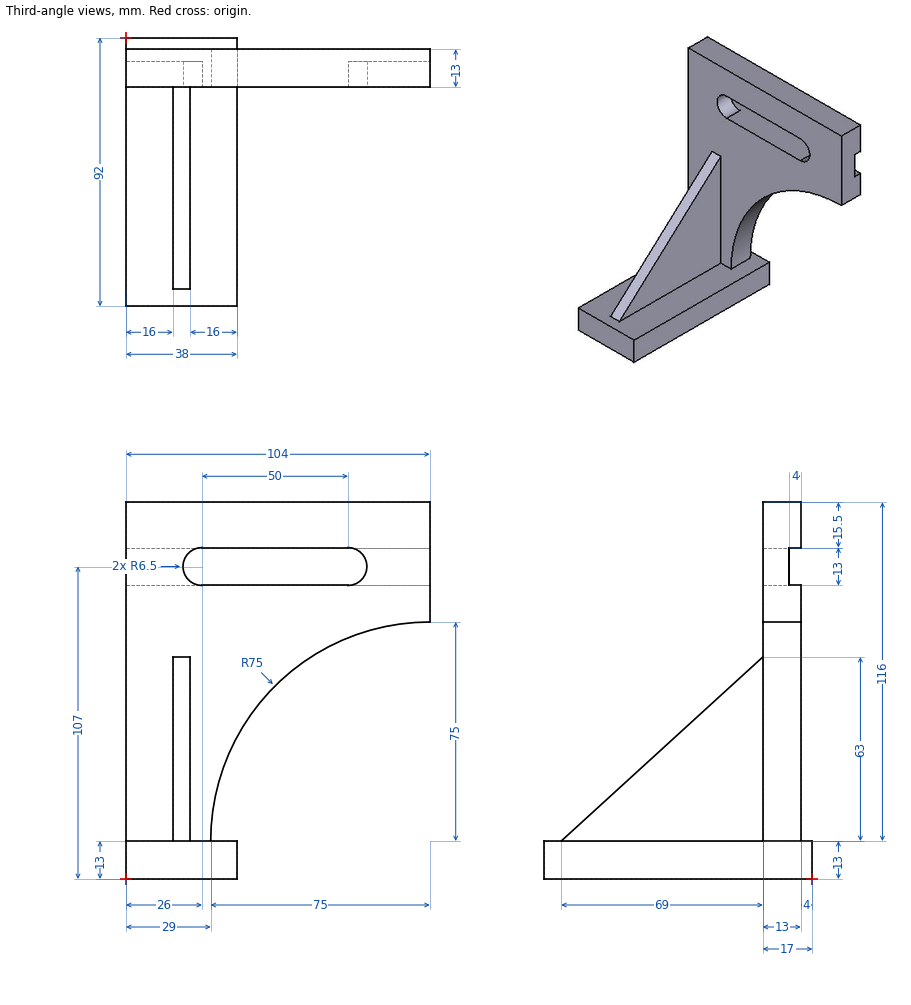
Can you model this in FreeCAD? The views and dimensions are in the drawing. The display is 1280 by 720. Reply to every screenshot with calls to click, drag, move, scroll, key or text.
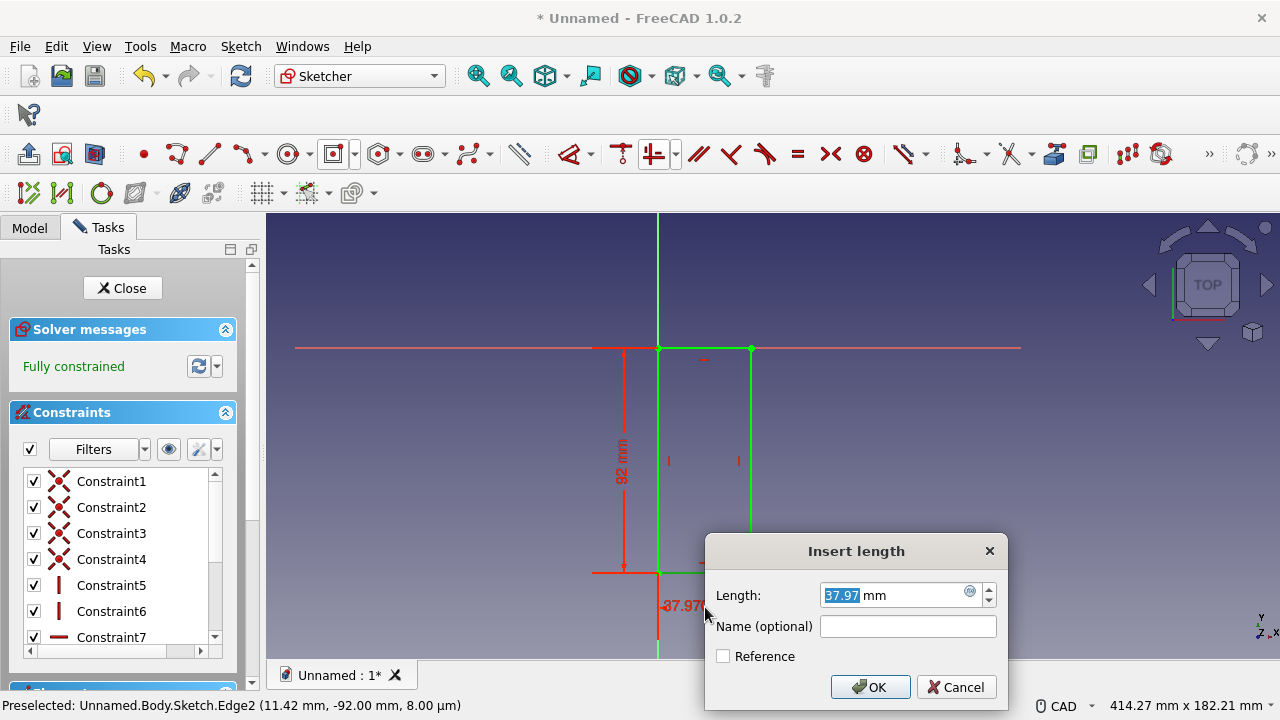
text(38)
key(Return)
key(Escape)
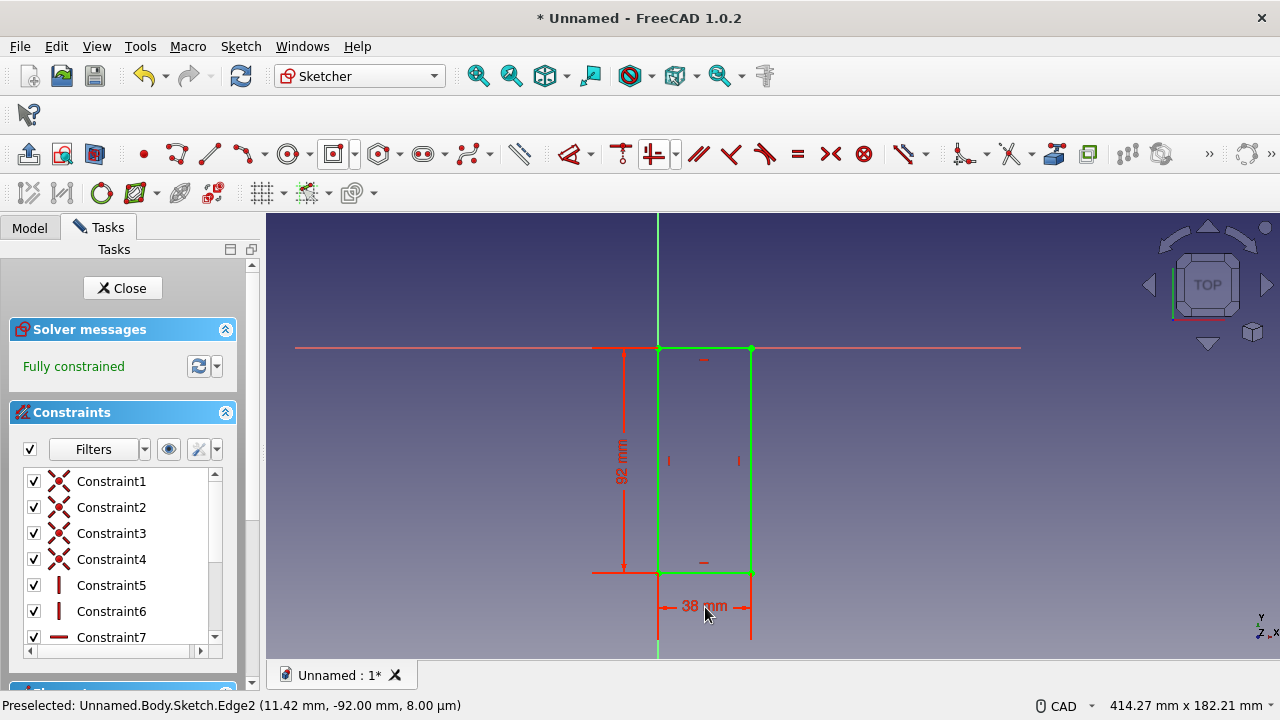
click(123, 288)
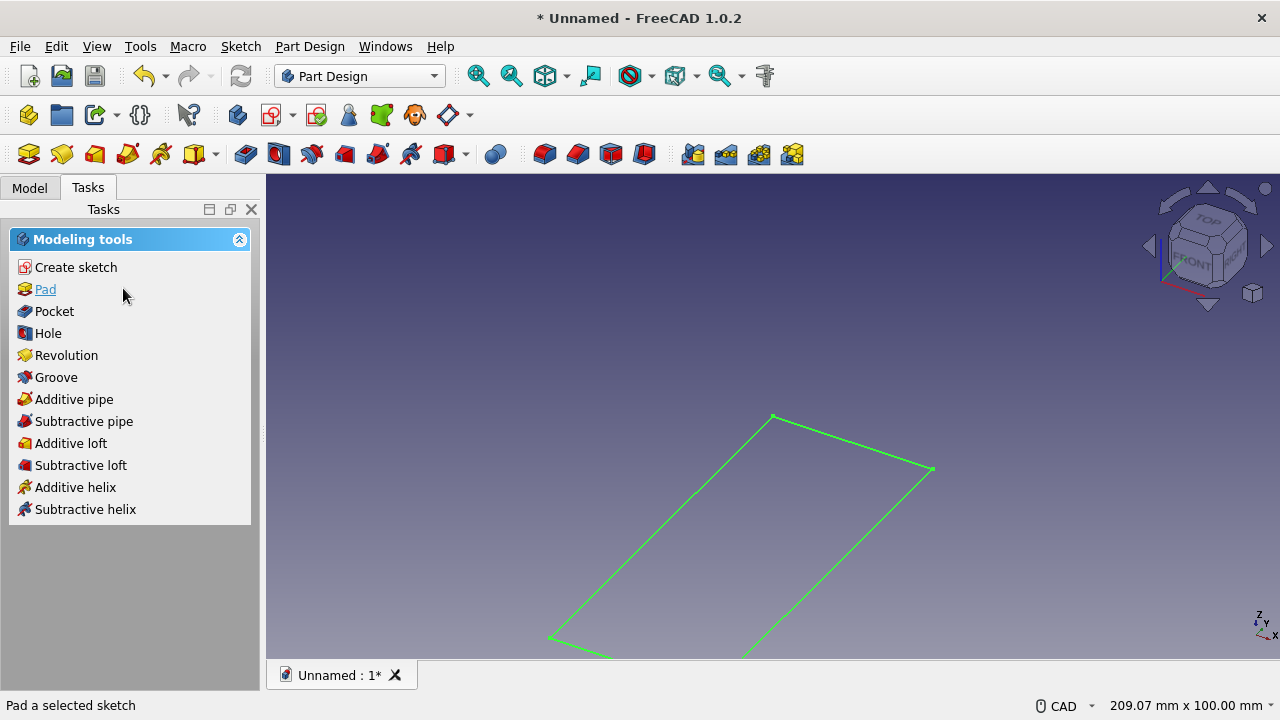
click(29, 154)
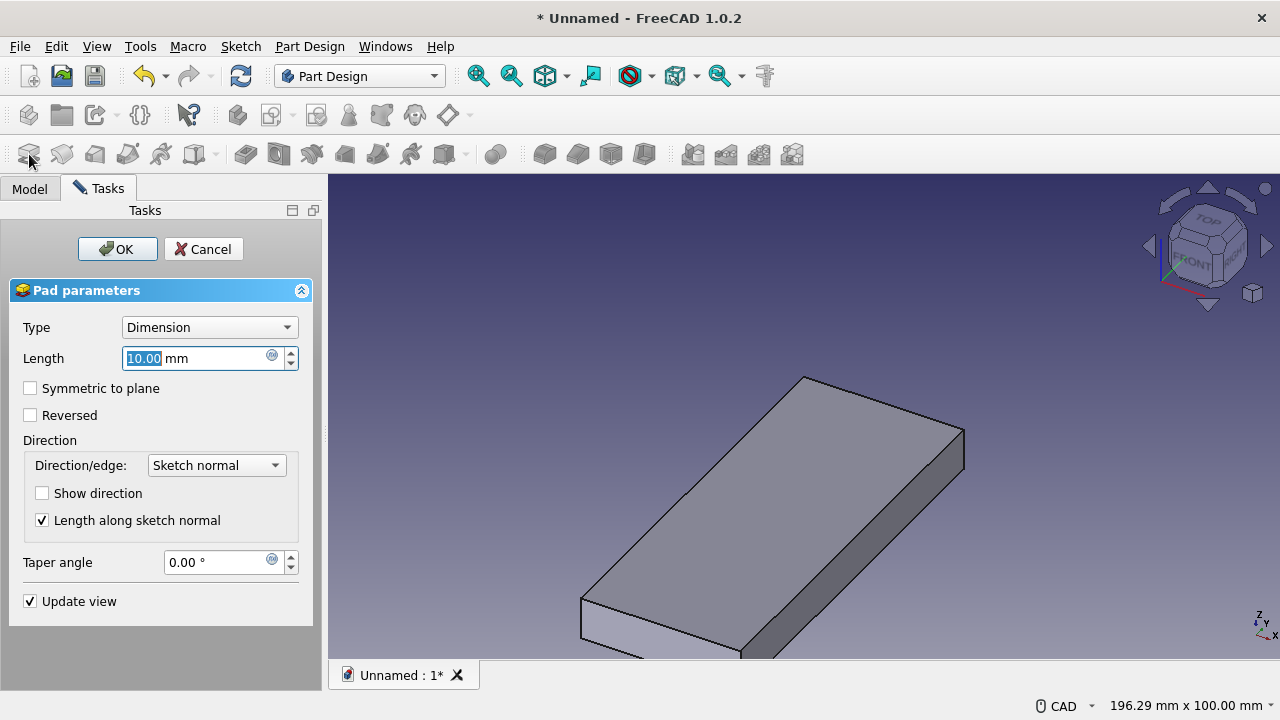
text(13)
key(Tab)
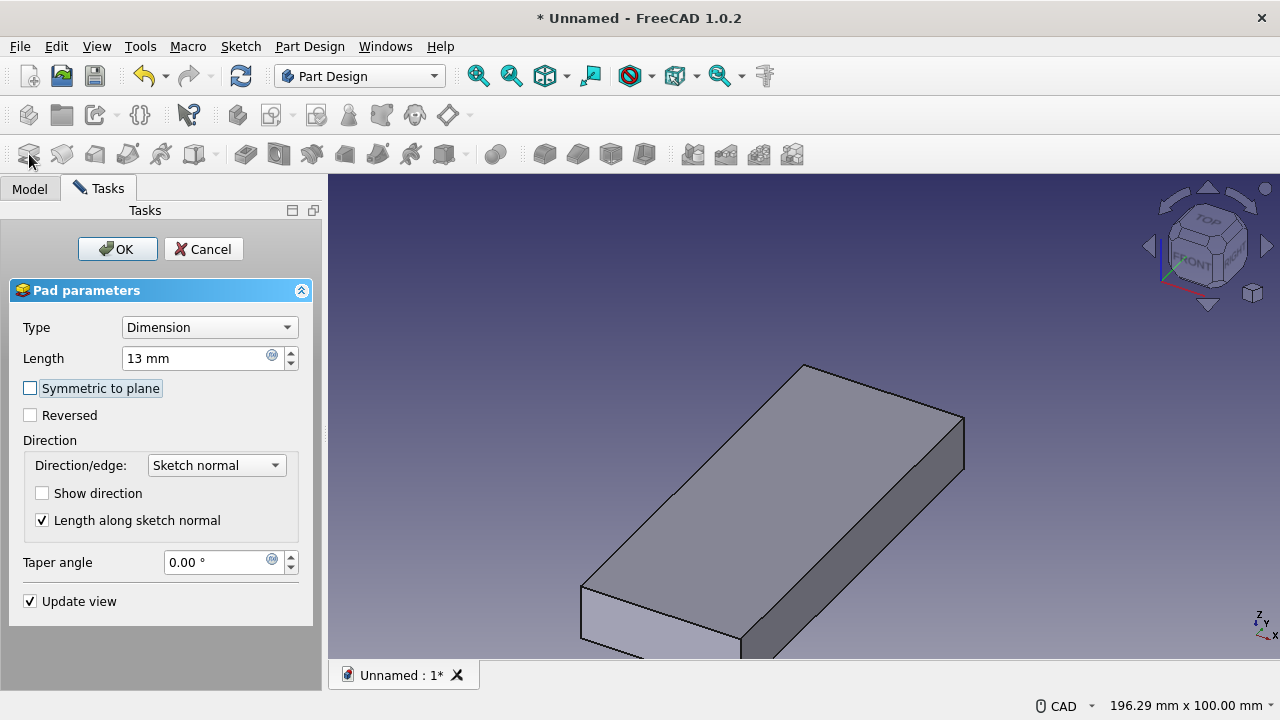
click(118, 249)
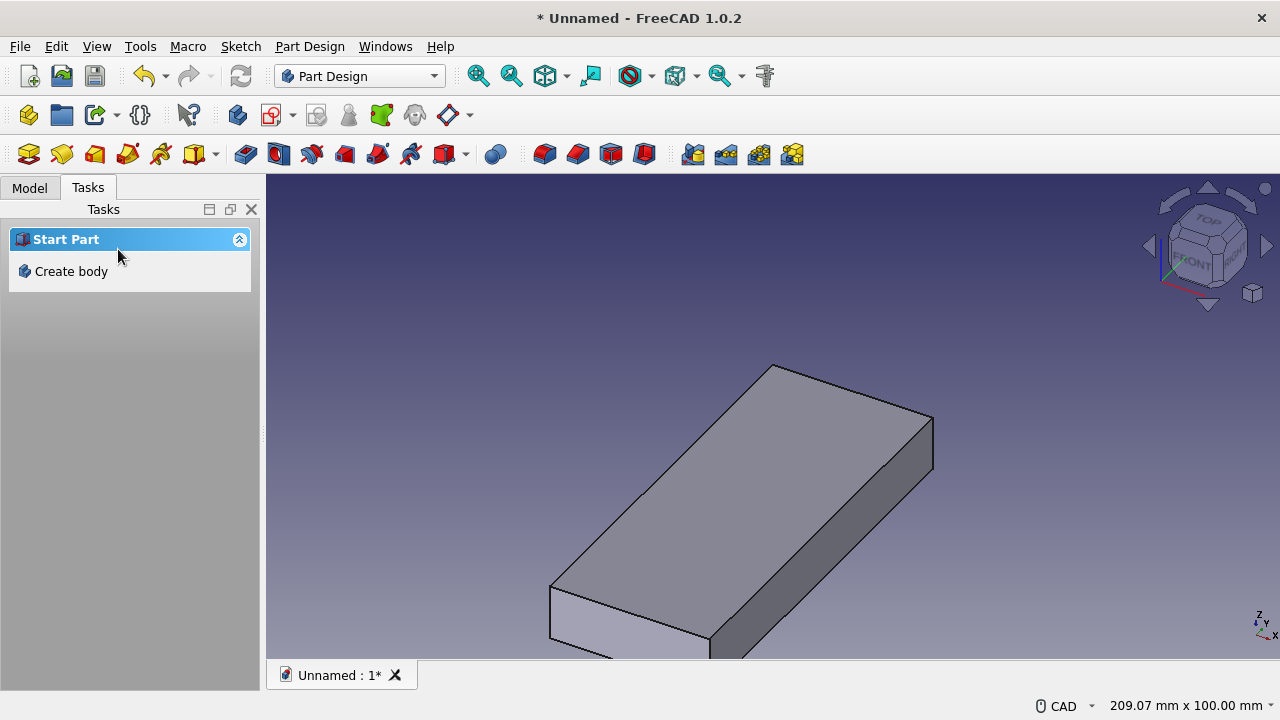
key(v)
key(f)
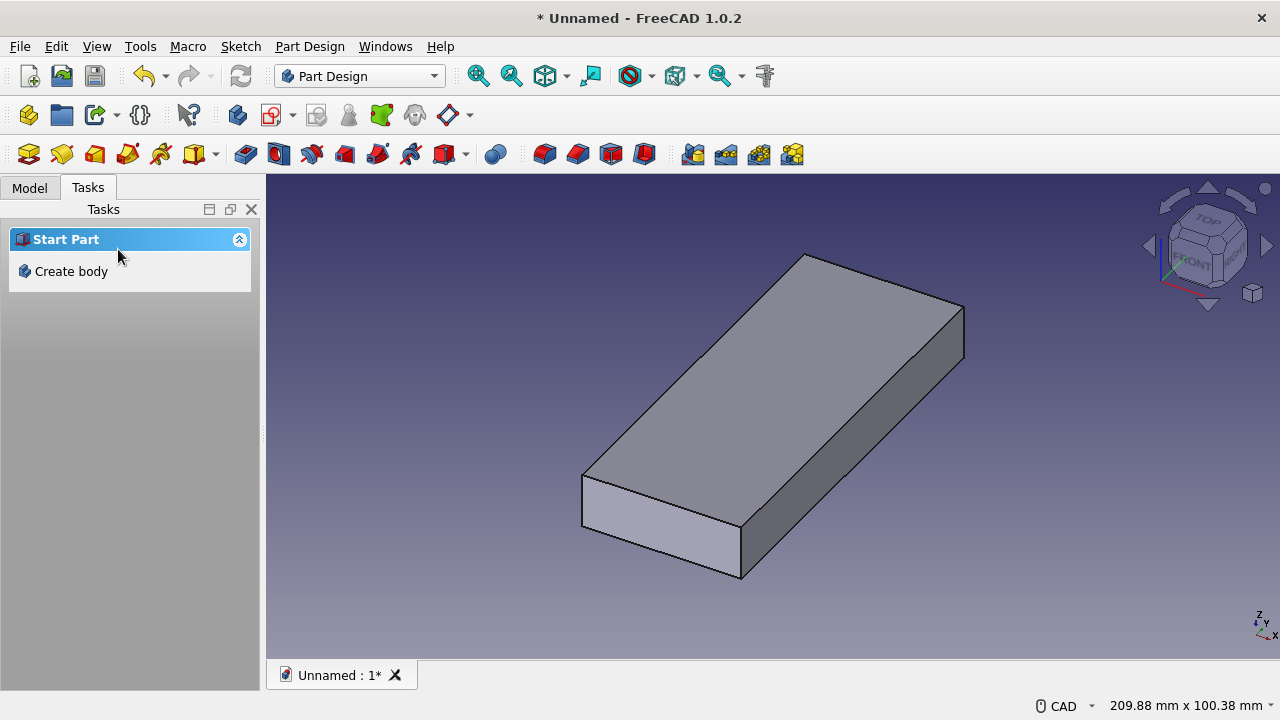
key(6)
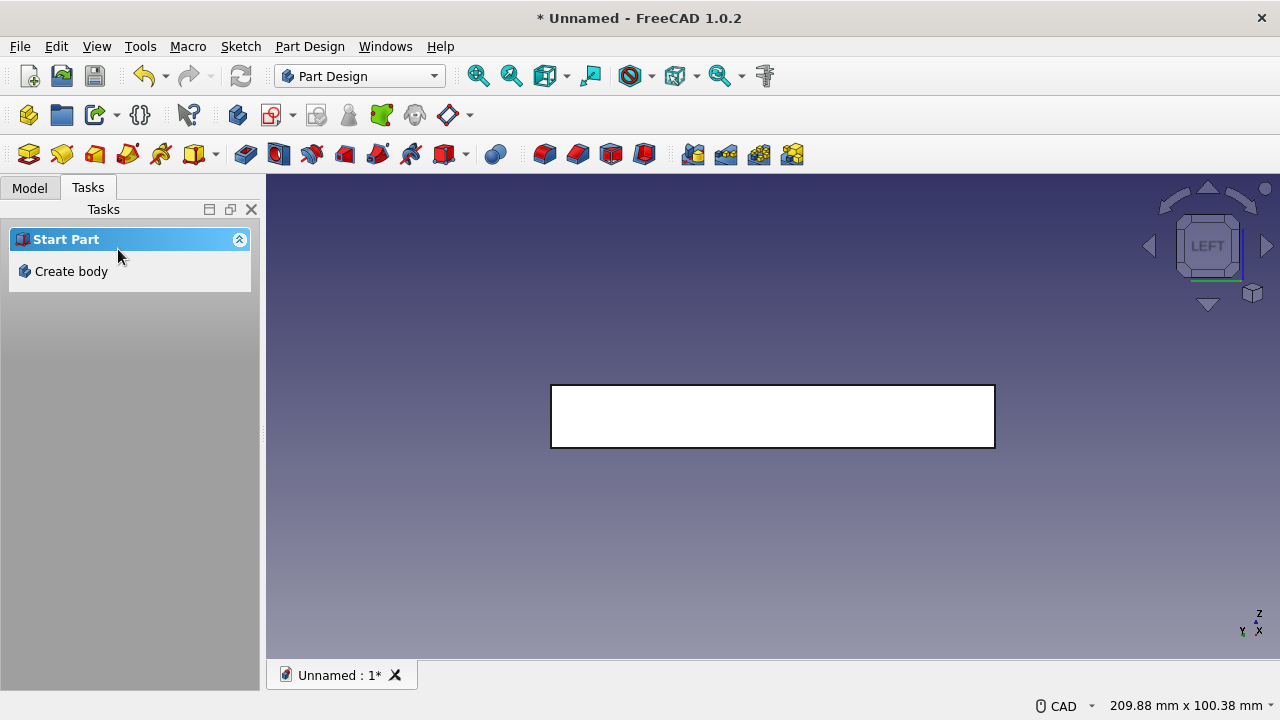
click(479, 76)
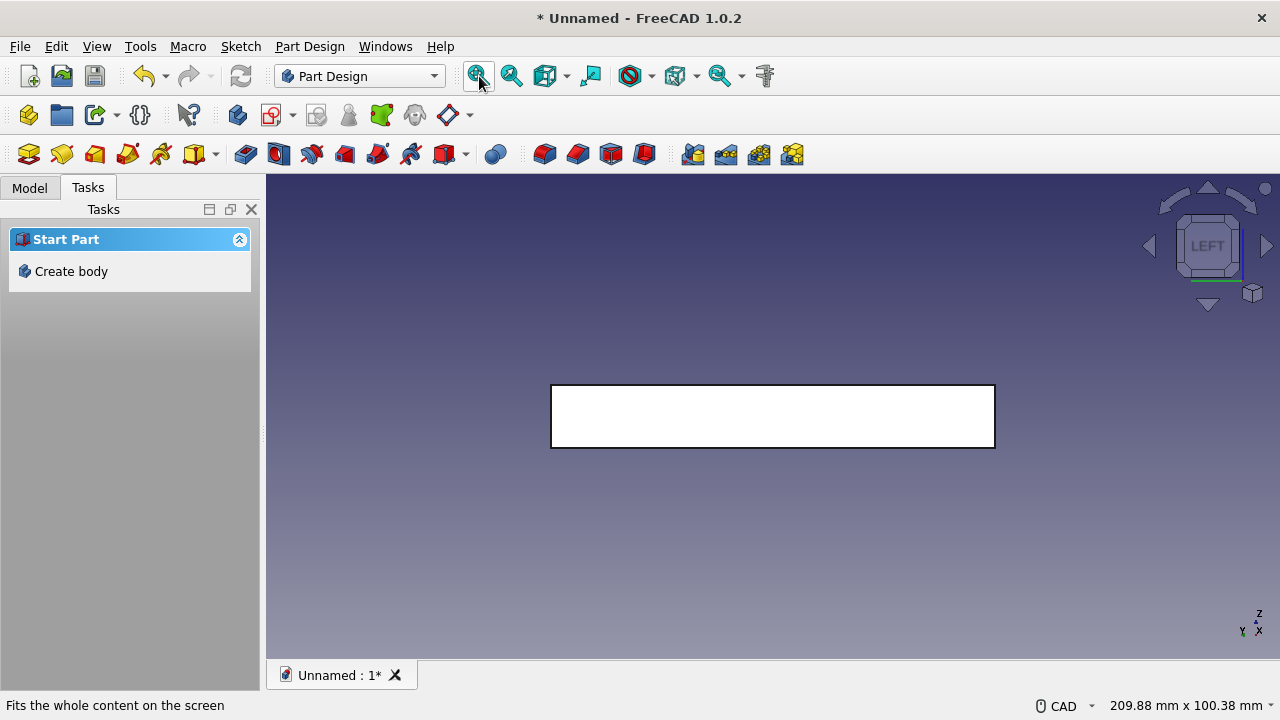
click(583, 415)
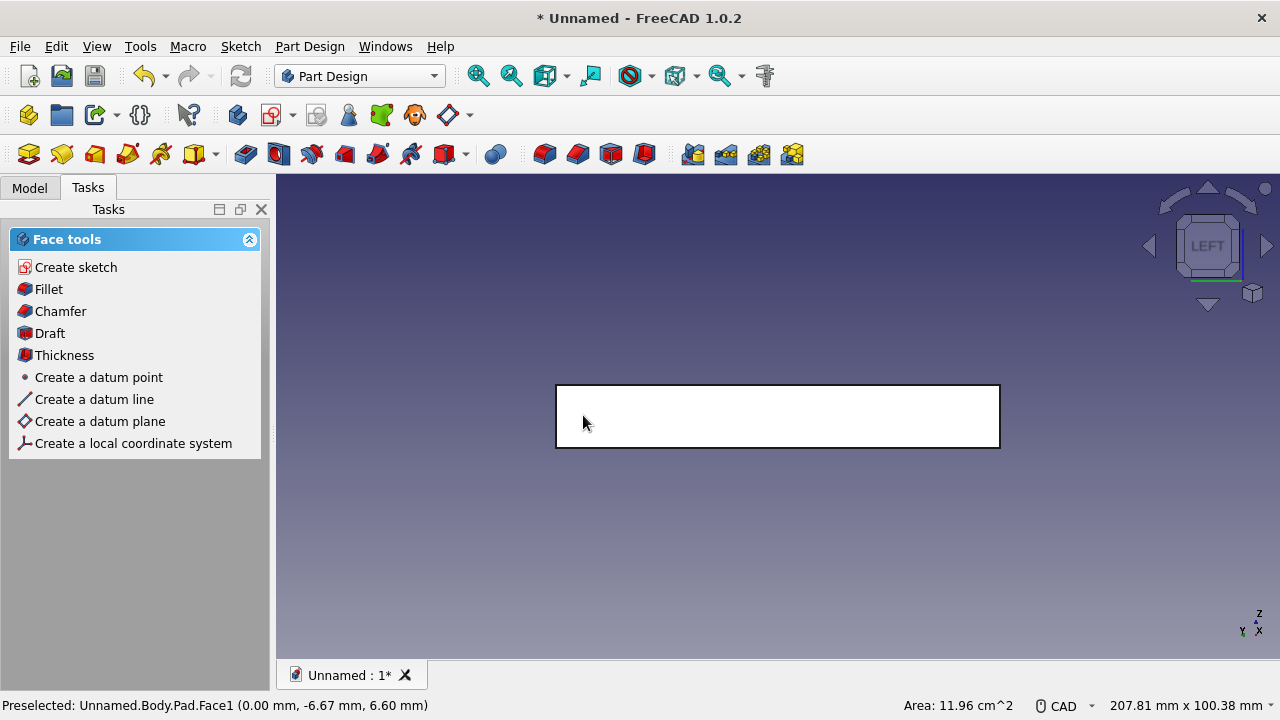
click(270, 116)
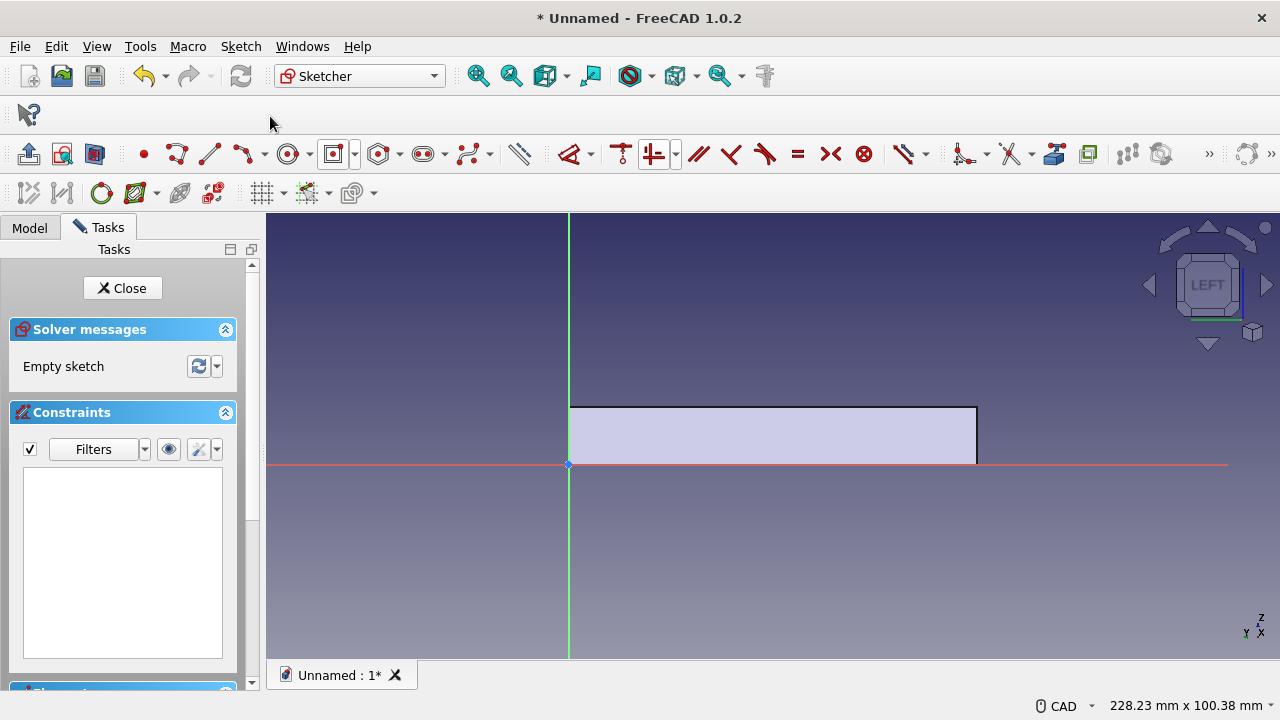
scroll(785, 631, down, 4)